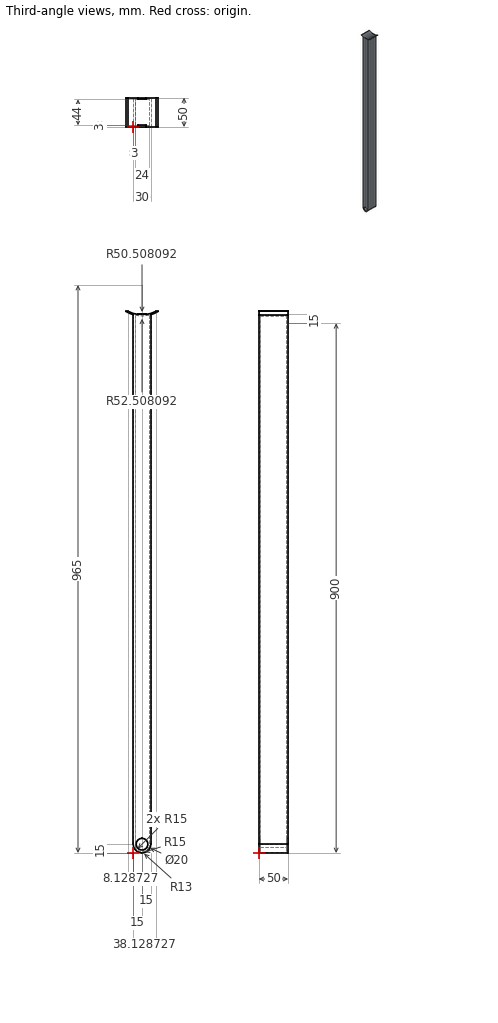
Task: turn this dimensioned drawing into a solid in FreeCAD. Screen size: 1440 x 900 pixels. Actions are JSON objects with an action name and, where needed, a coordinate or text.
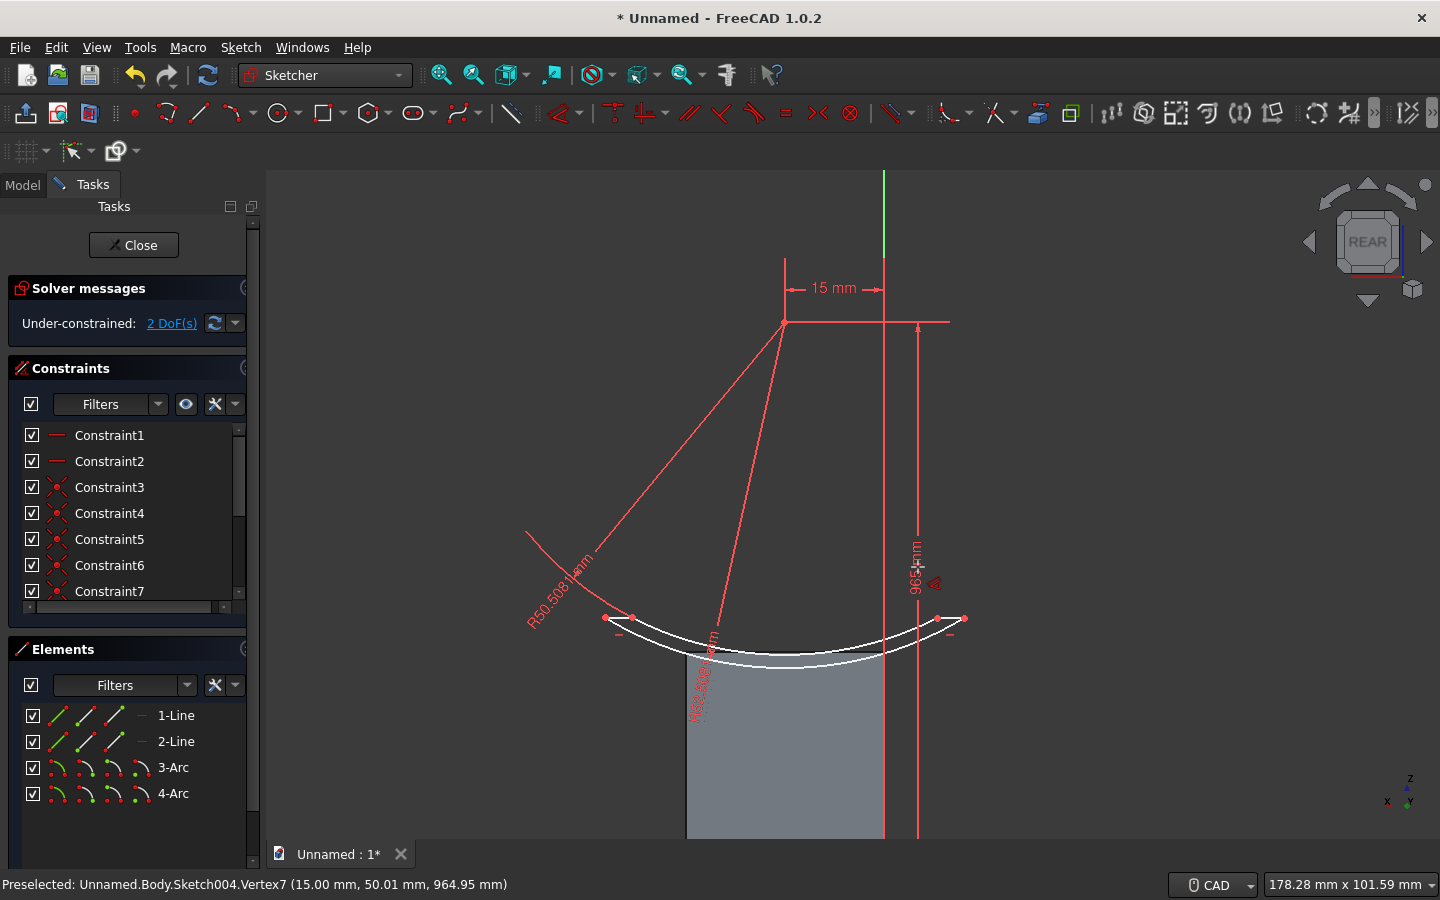
{"action": "left_click", "coordinate": [937, 618]}
{"action": "left_click", "coordinate": [910, 536]}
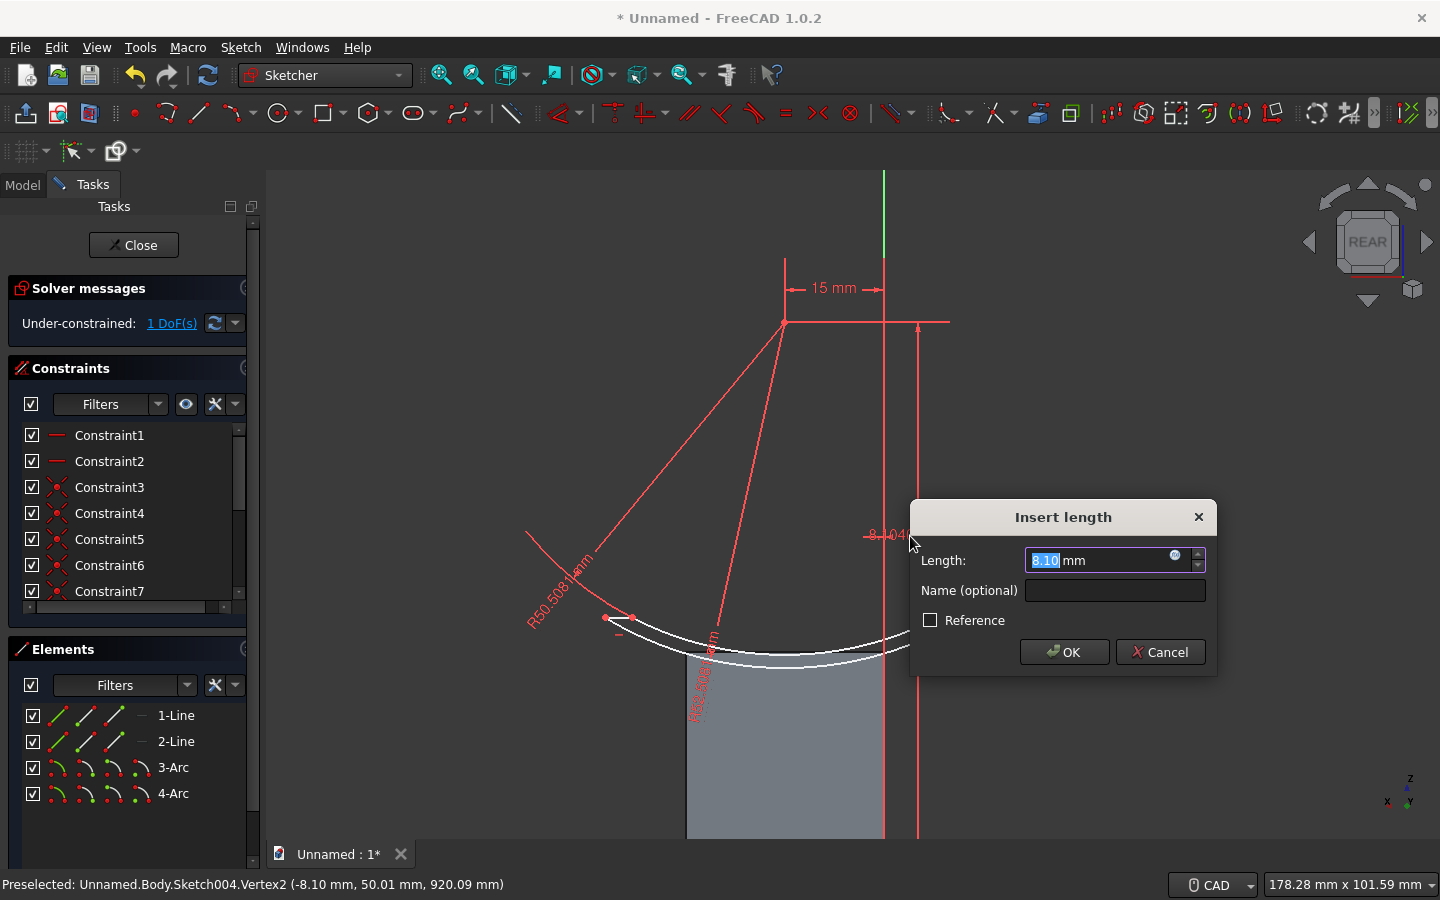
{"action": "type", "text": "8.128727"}
{"action": "key", "text": "Return"}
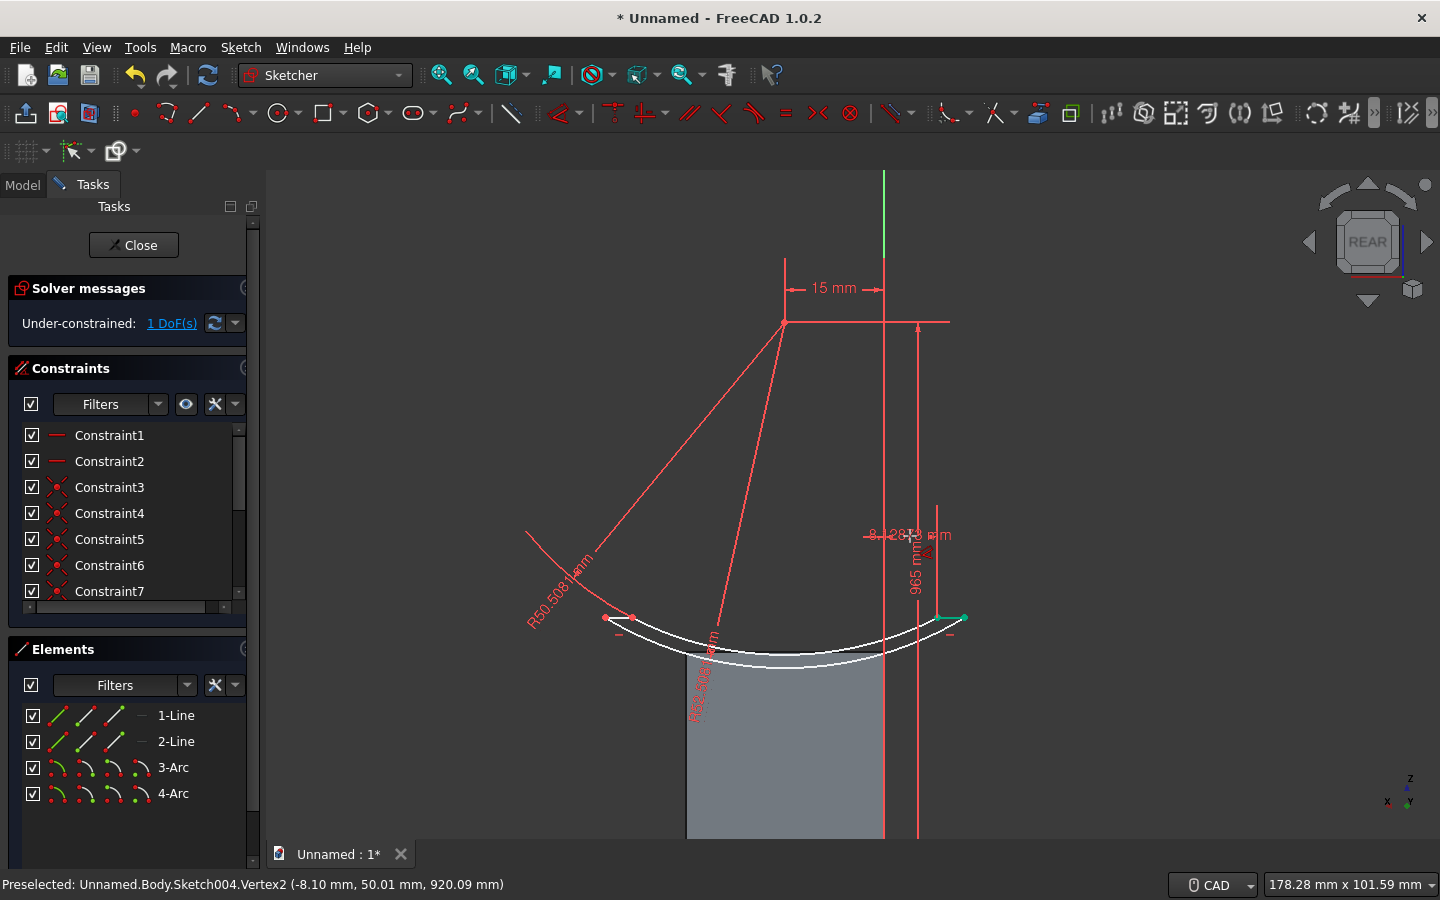
{"action": "left_click", "coordinate": [632, 618]}
{"action": "left_click", "coordinate": [758, 584]}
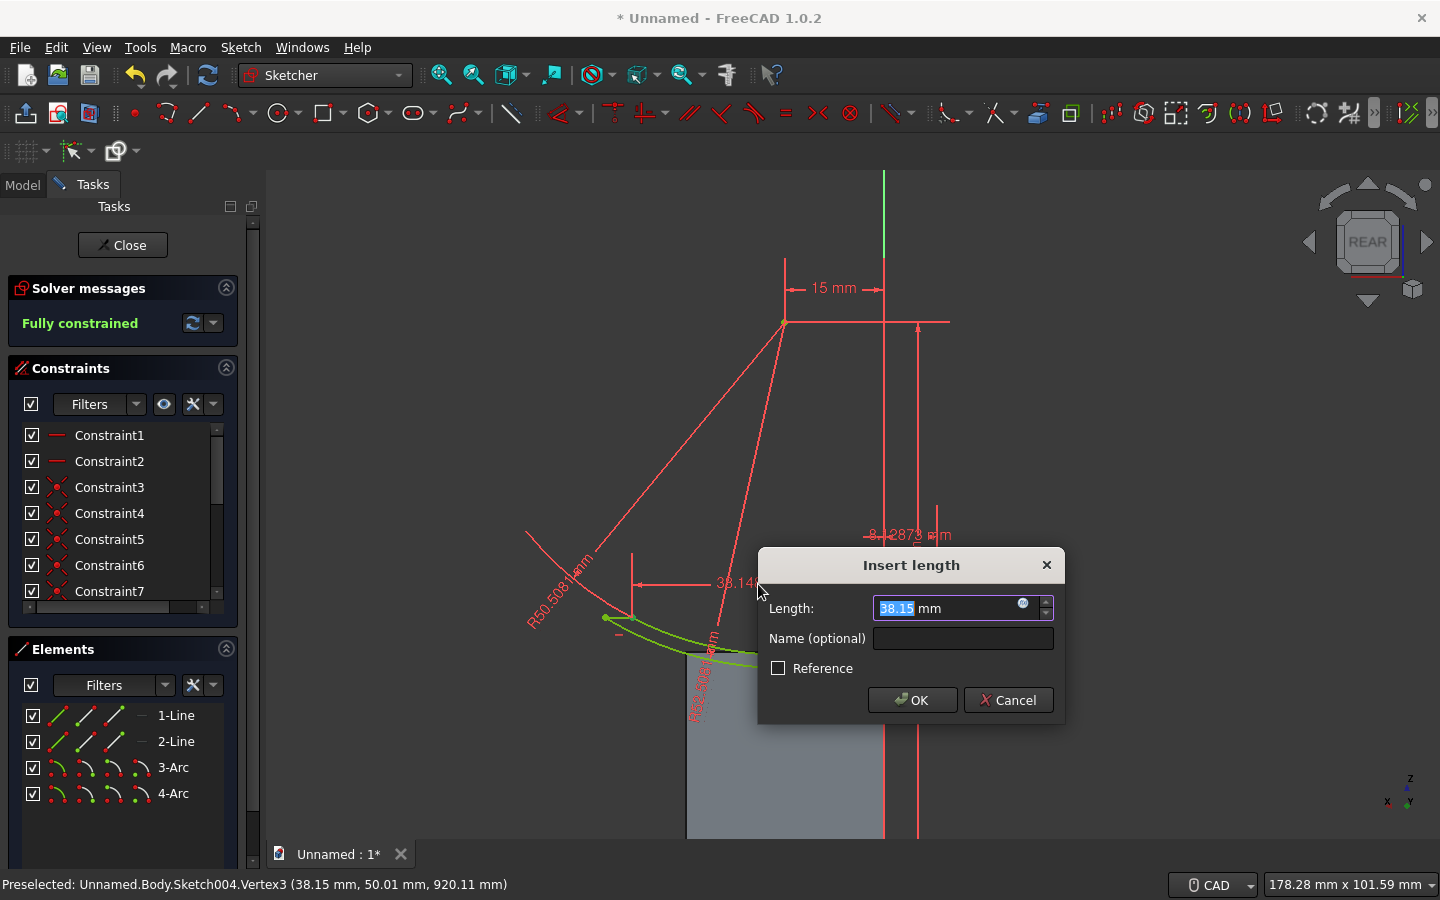
{"action": "type", "text": "38.128727"}
{"action": "key", "text": "Return"}
{"action": "key", "text": "Escape"}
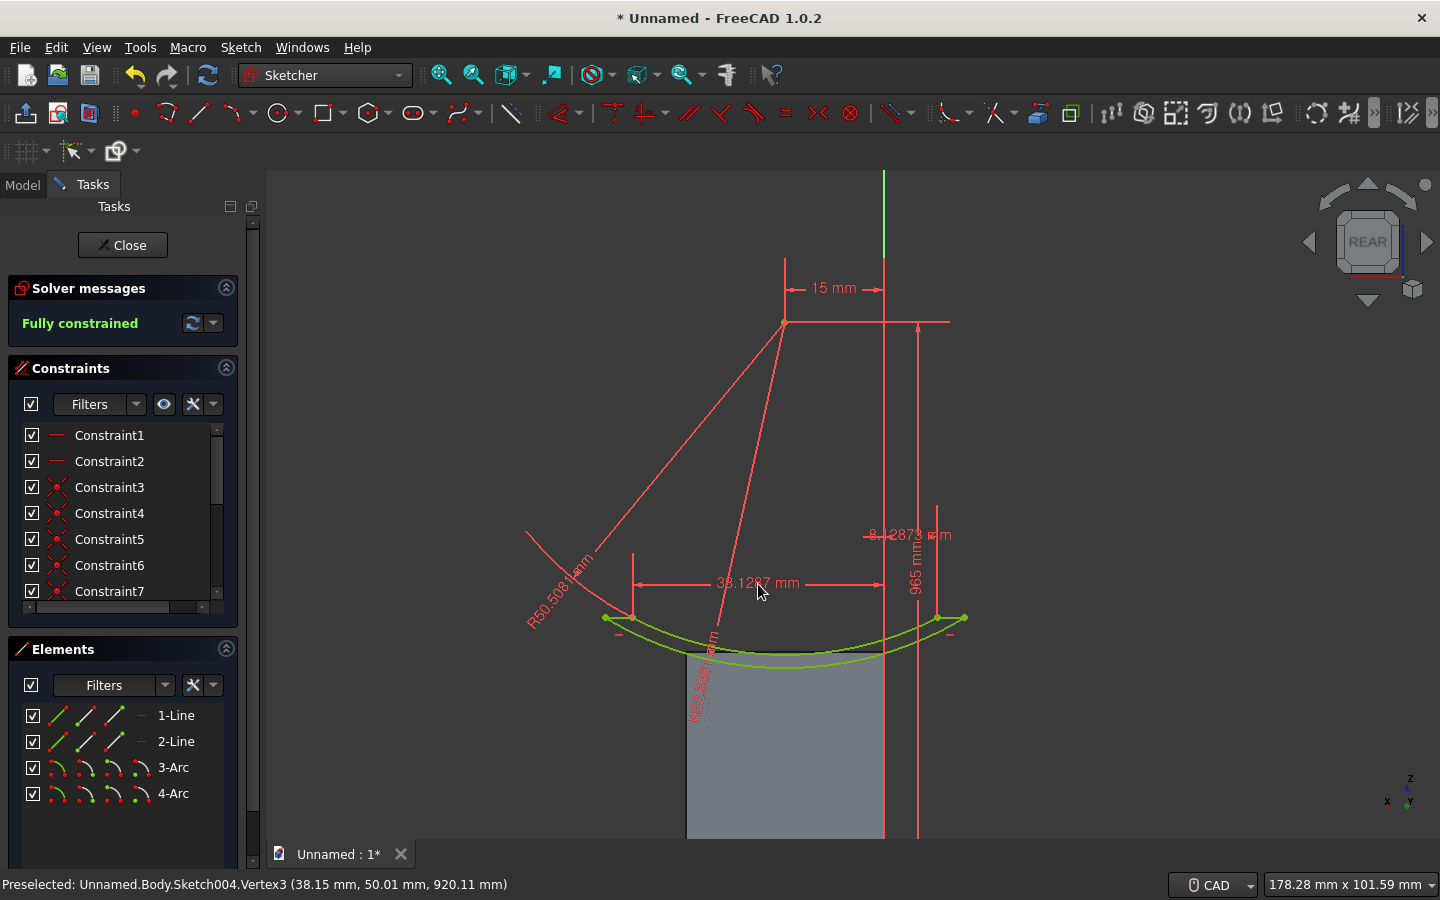
{"action": "left_click", "coordinate": [123, 245]}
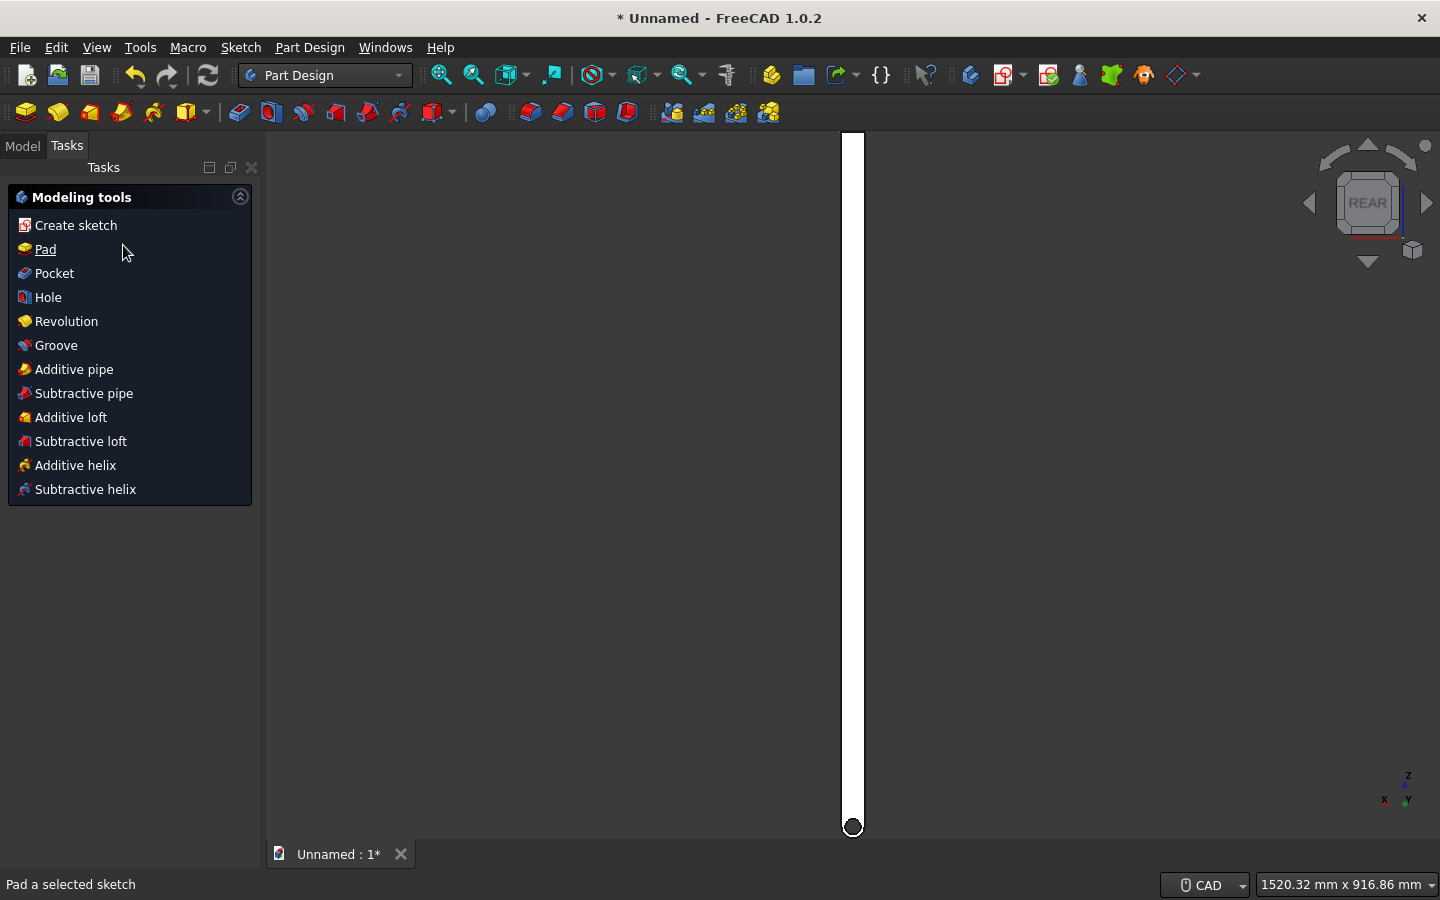
{"action": "left_click", "coordinate": [26, 112]}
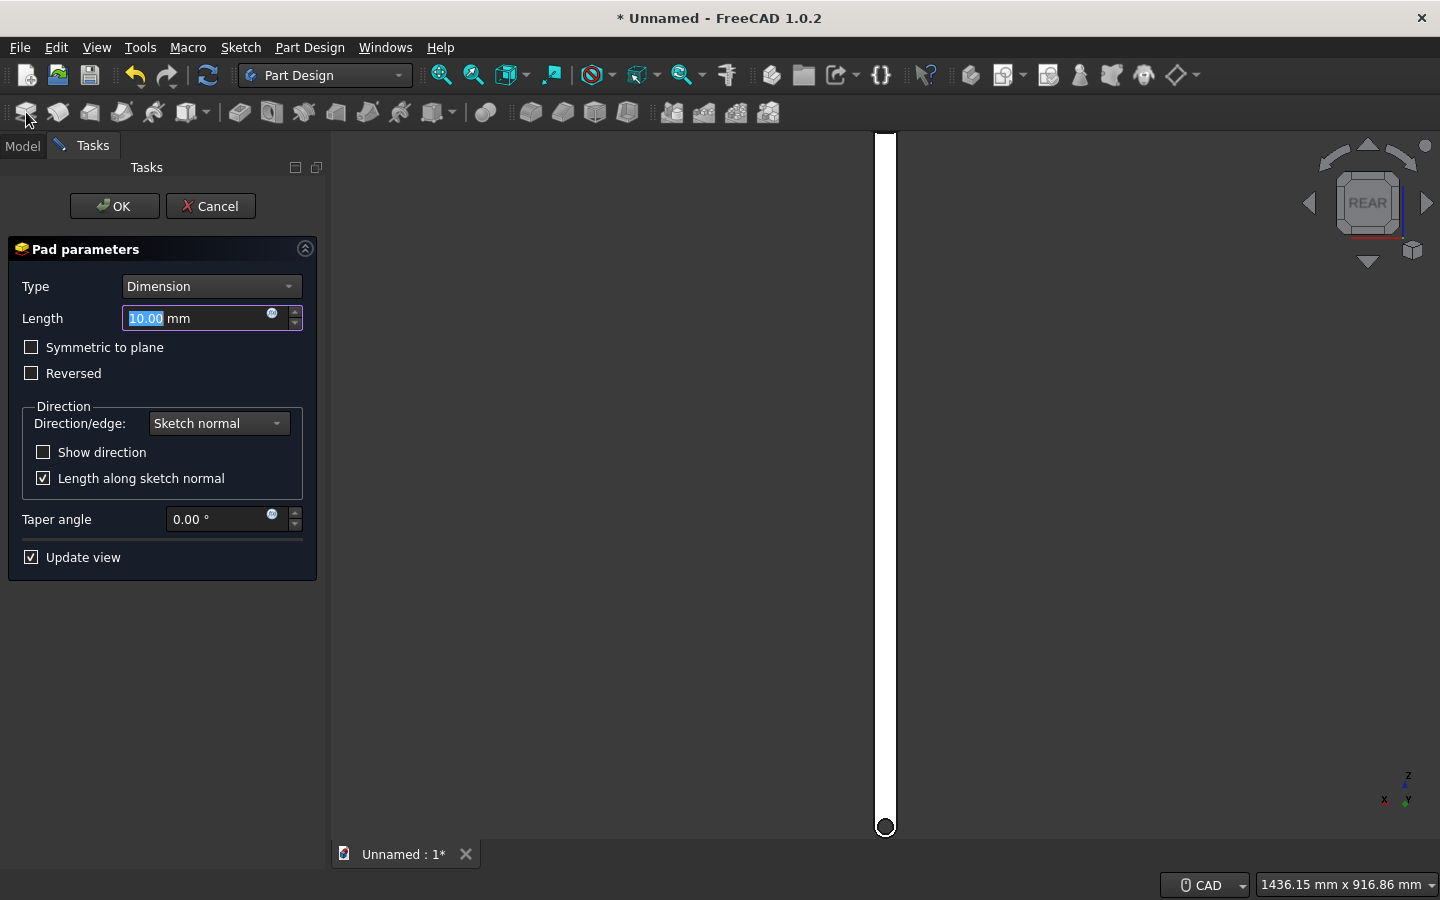
{"action": "type", "text": "50"}
{"action": "key", "text": "Tab"}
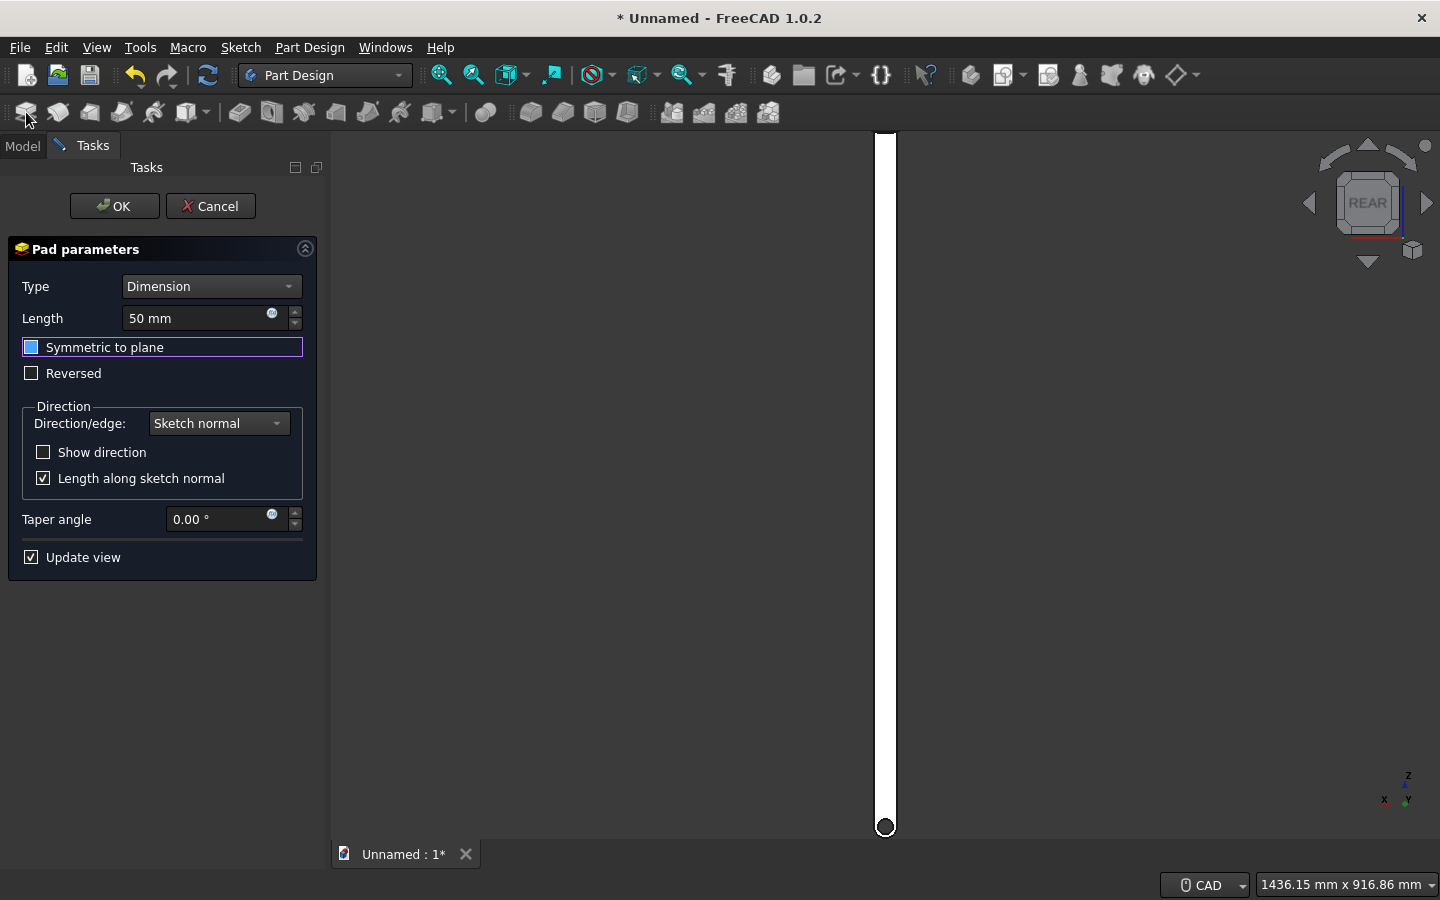
{"action": "left_click", "coordinate": [30, 373]}